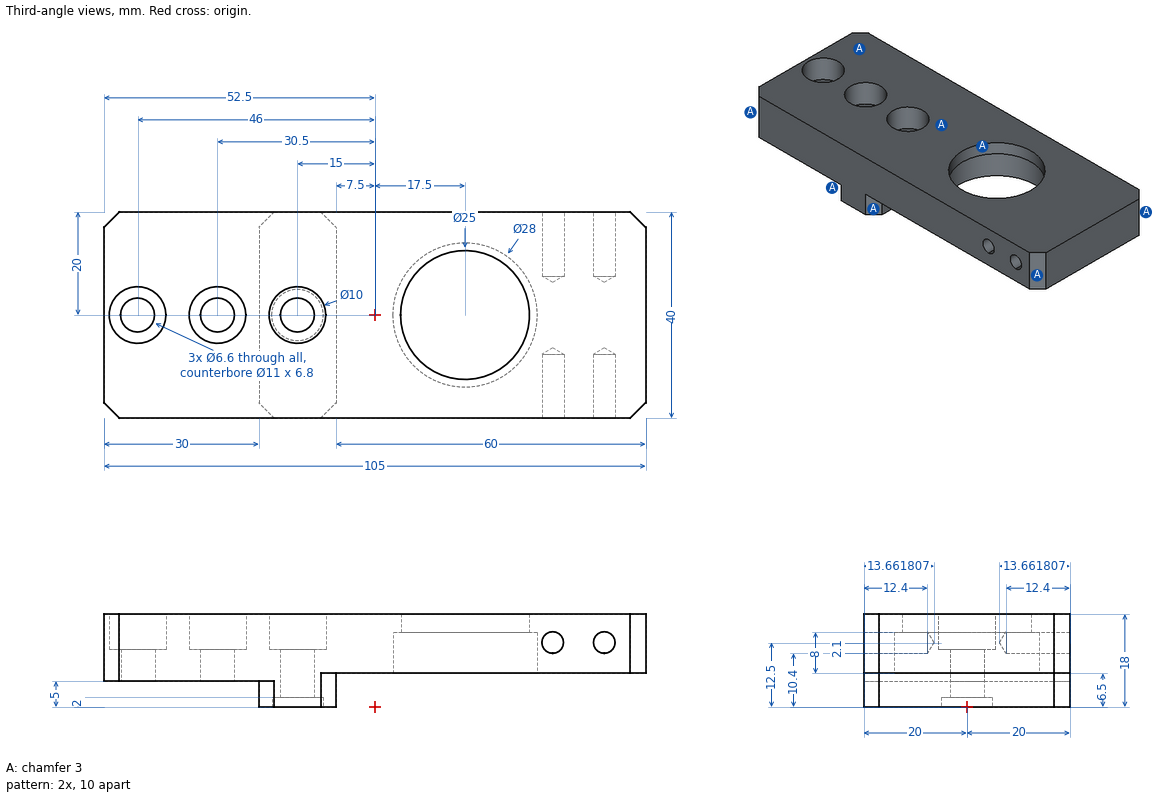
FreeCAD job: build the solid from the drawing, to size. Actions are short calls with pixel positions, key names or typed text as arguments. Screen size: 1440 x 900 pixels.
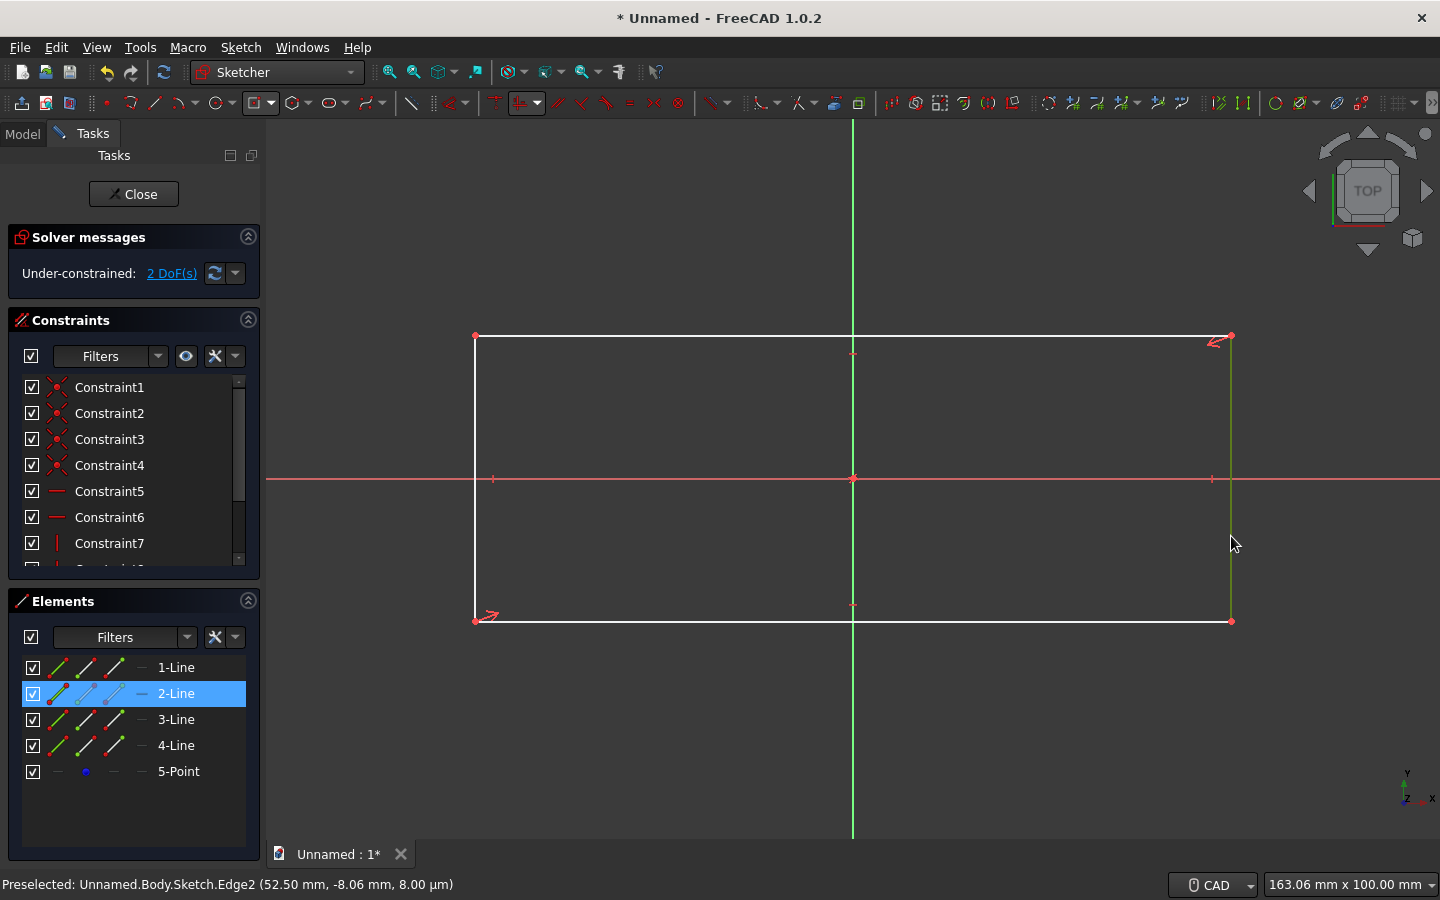
click(468, 104)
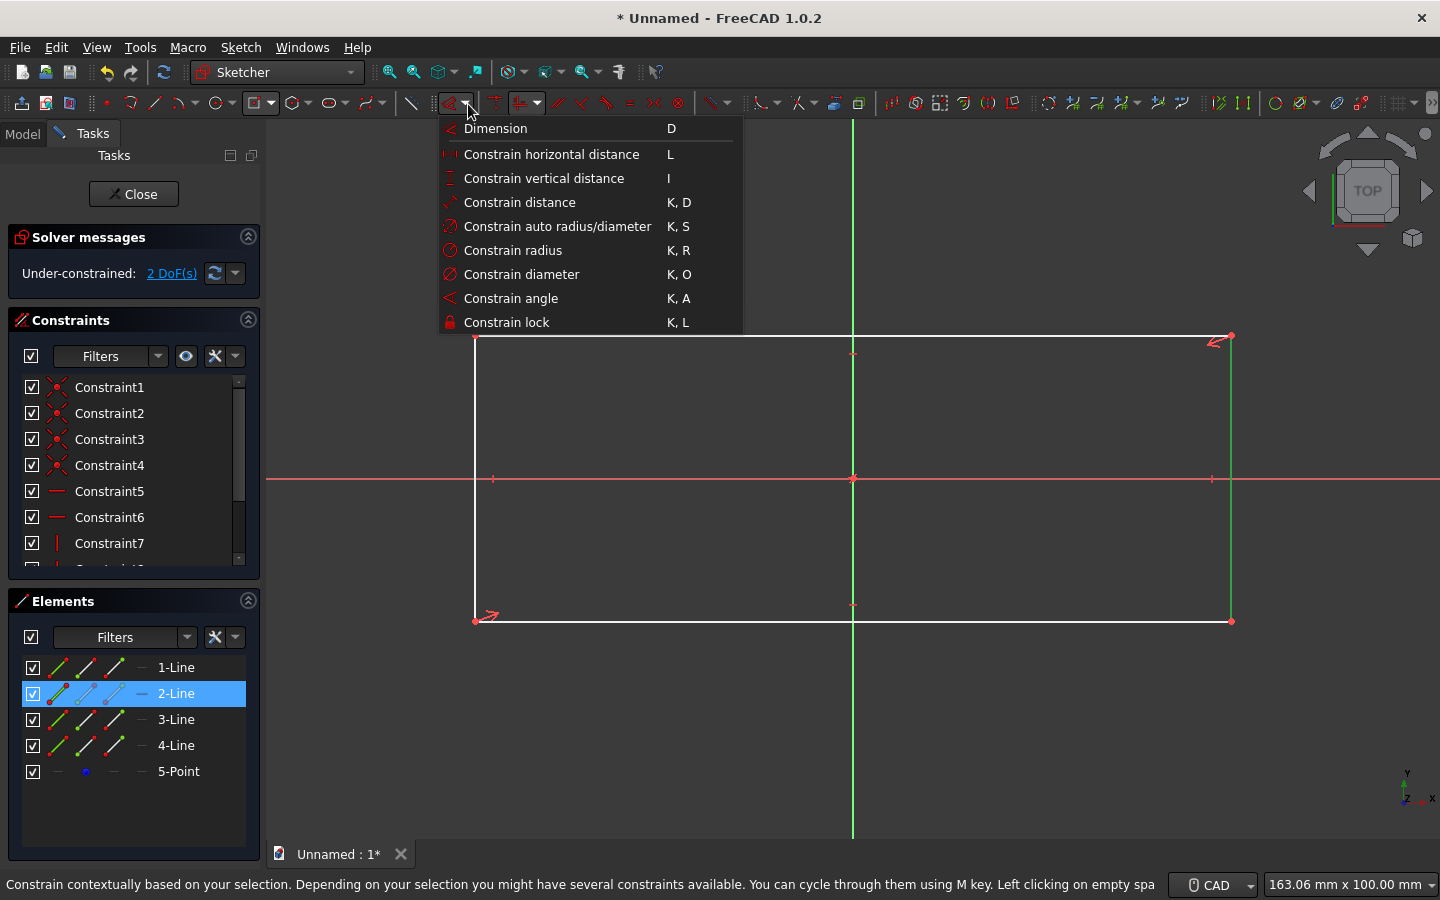
click(591, 178)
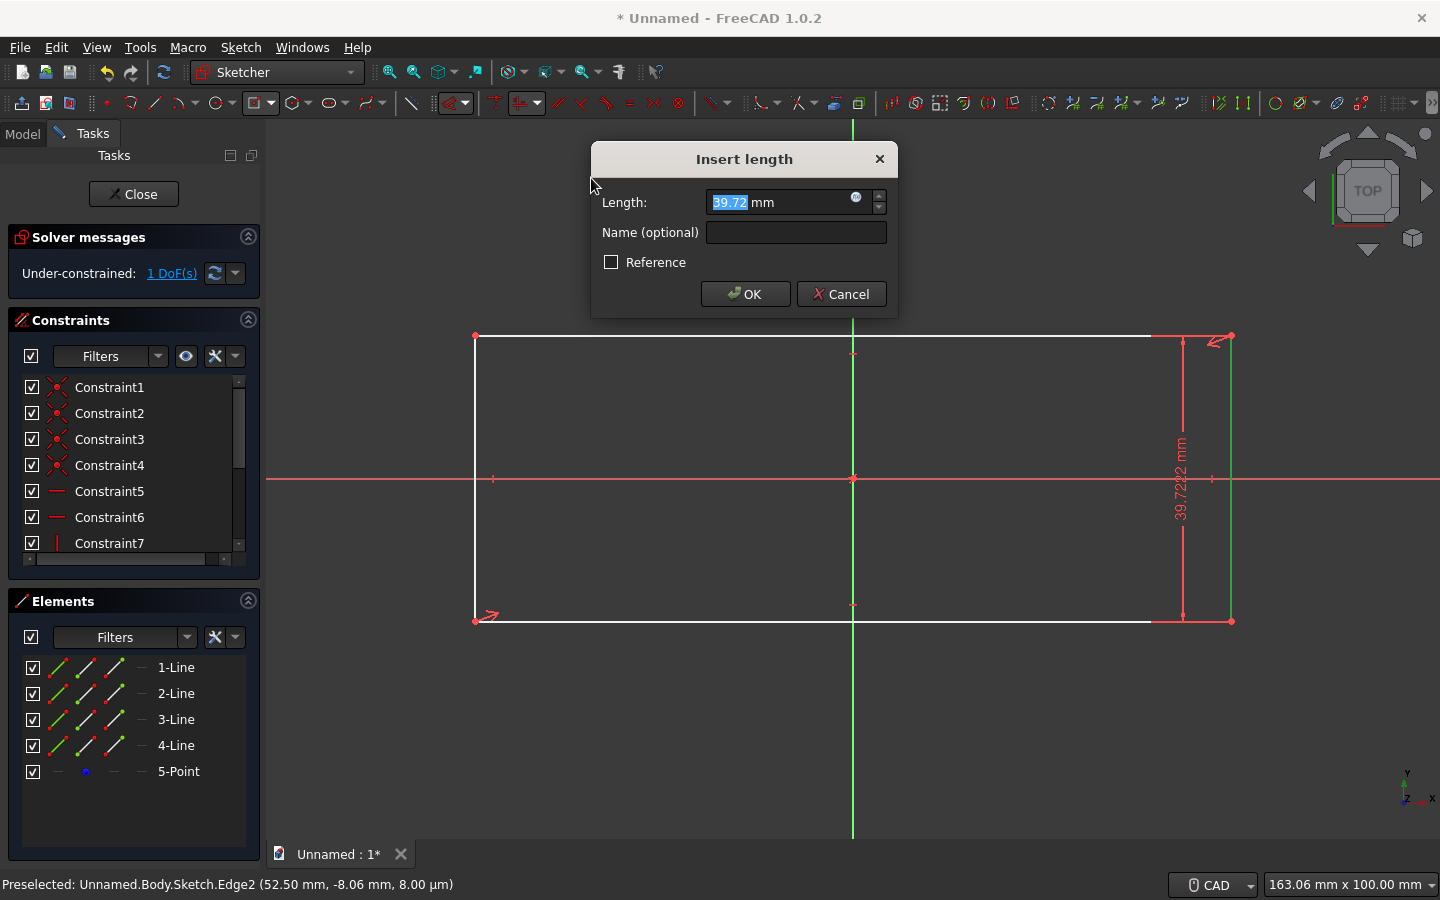
text(40)
key(Return)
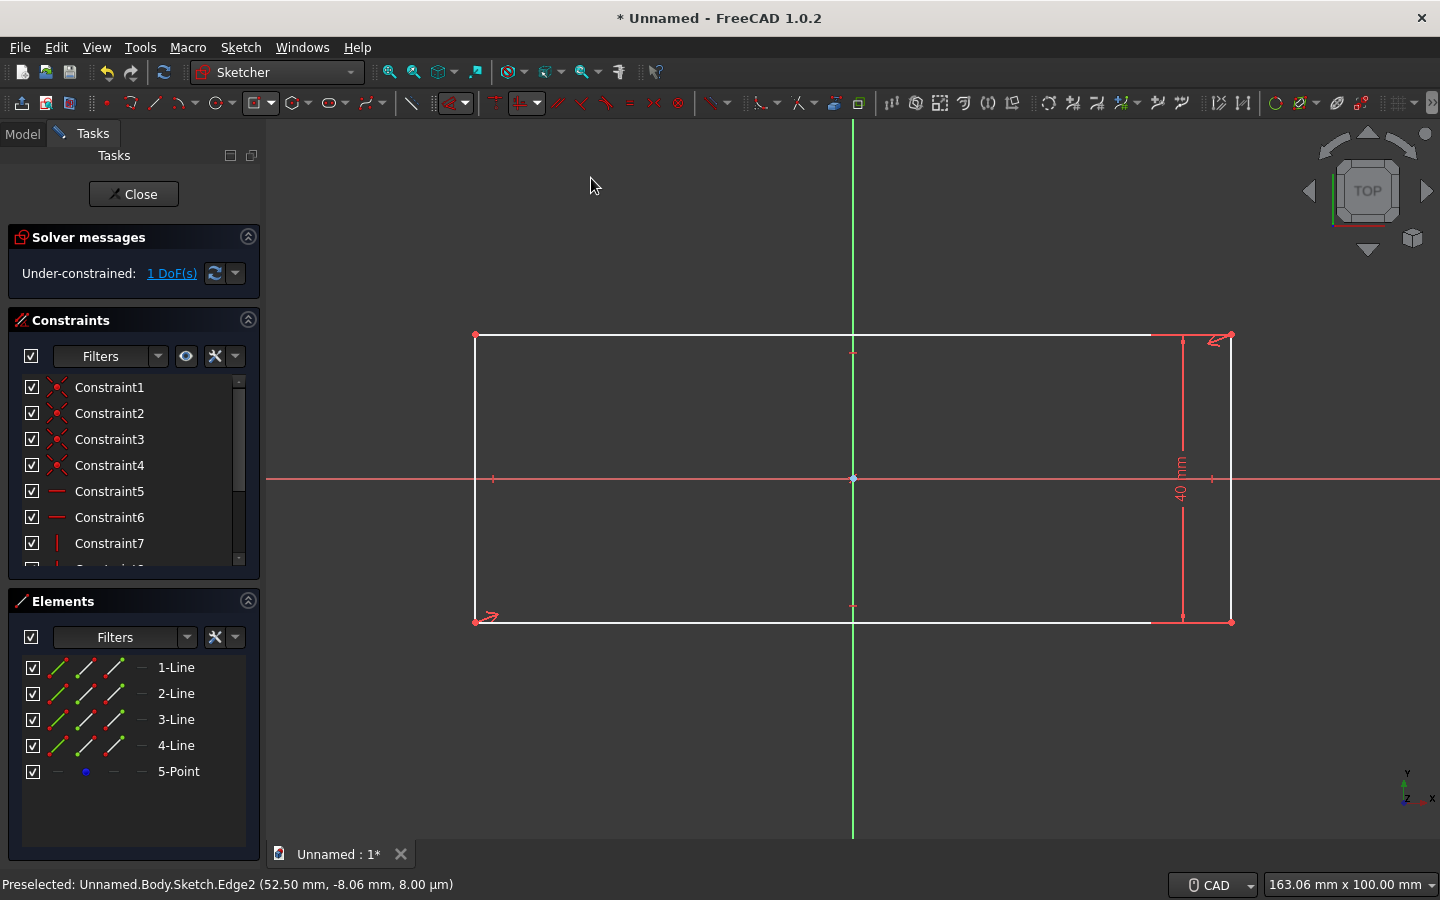
click(702, 623)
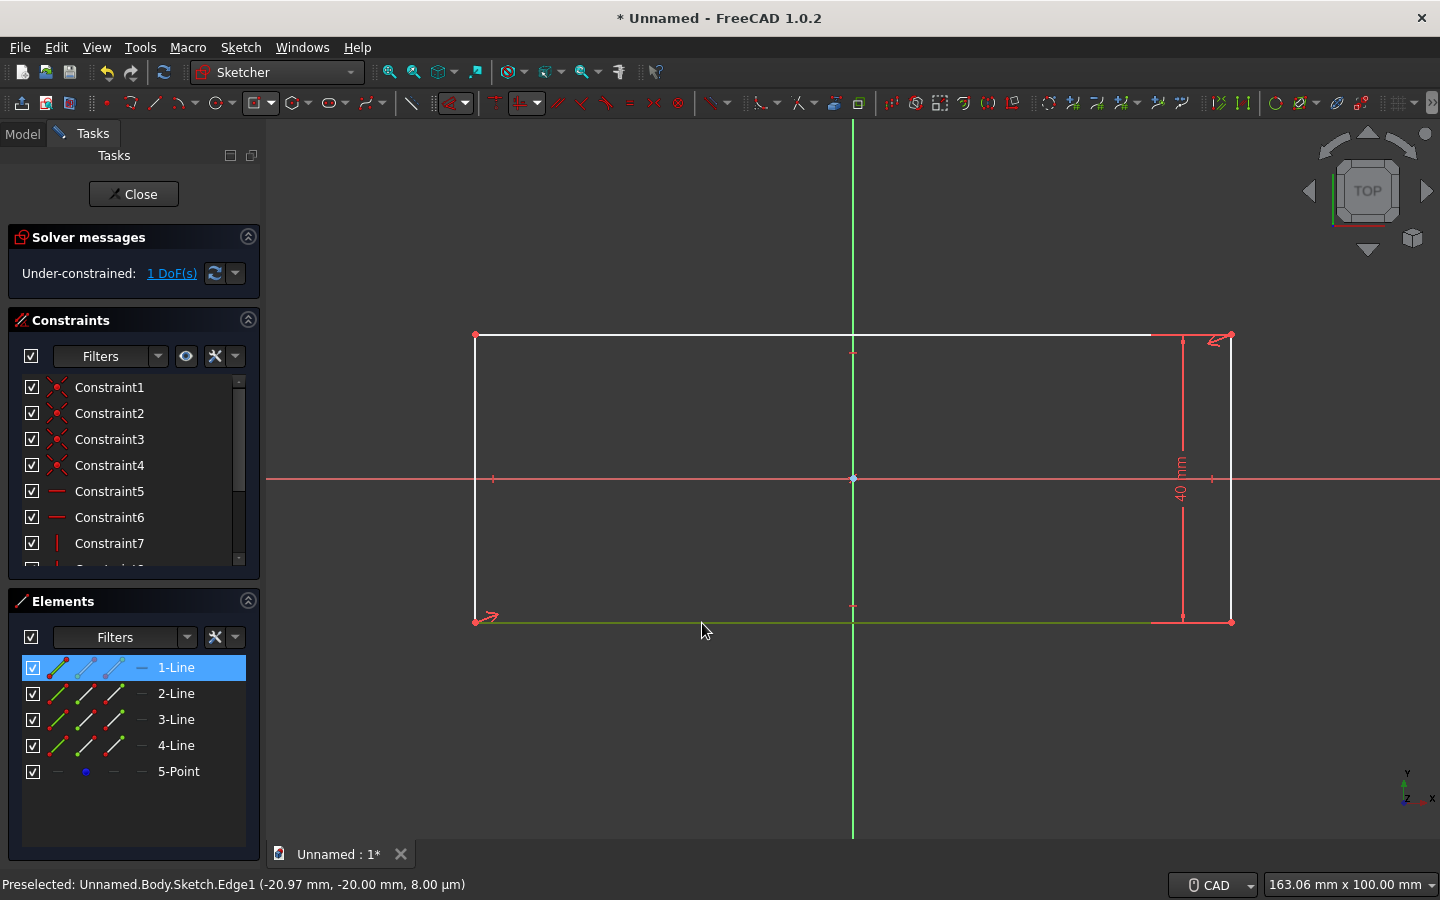
click(468, 104)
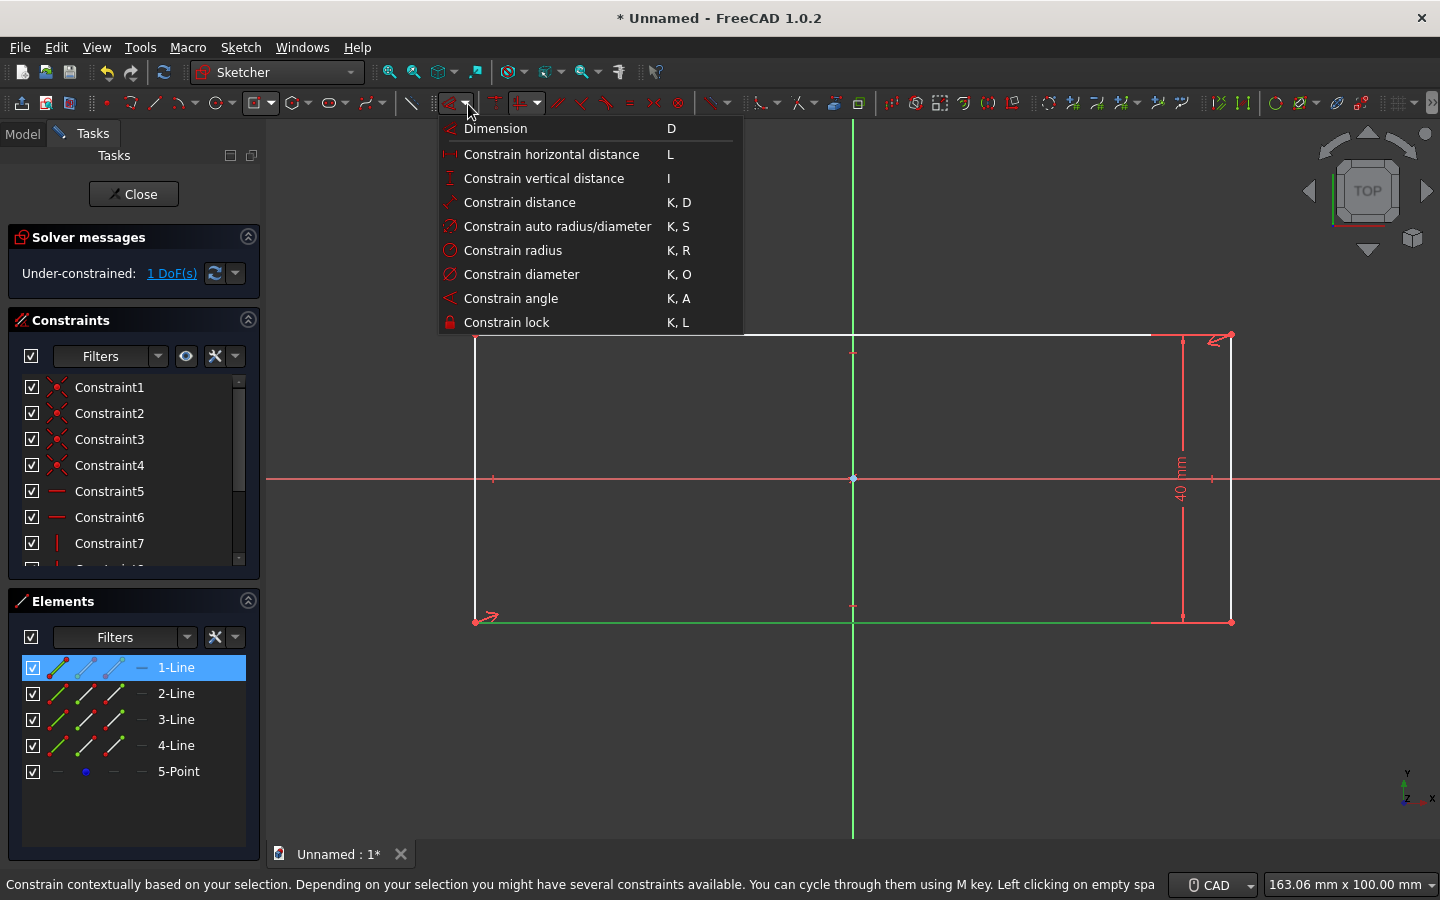
click(591, 154)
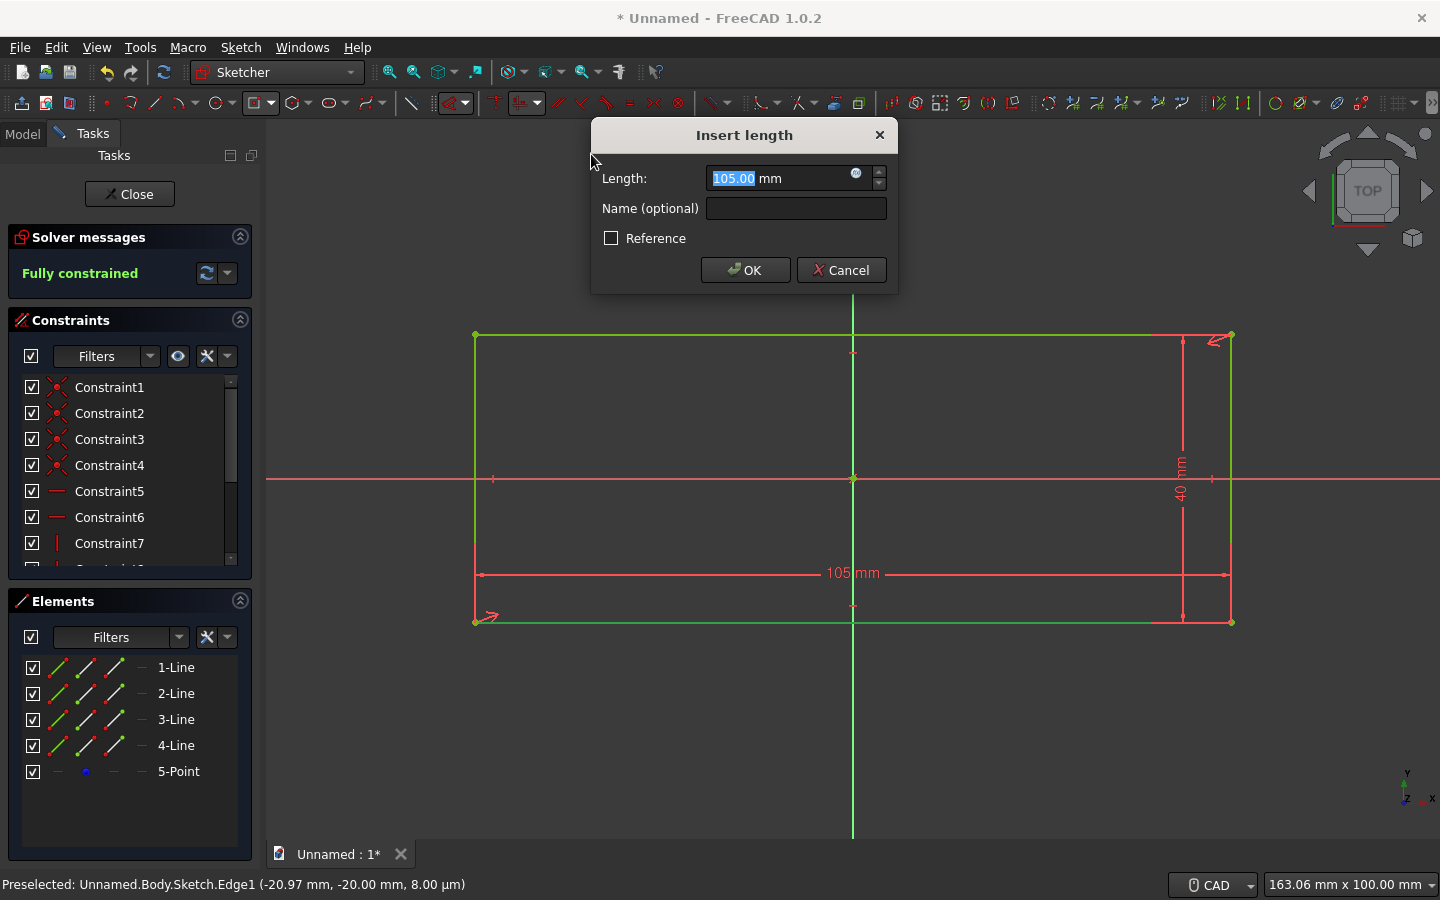
text(105)
key(Return)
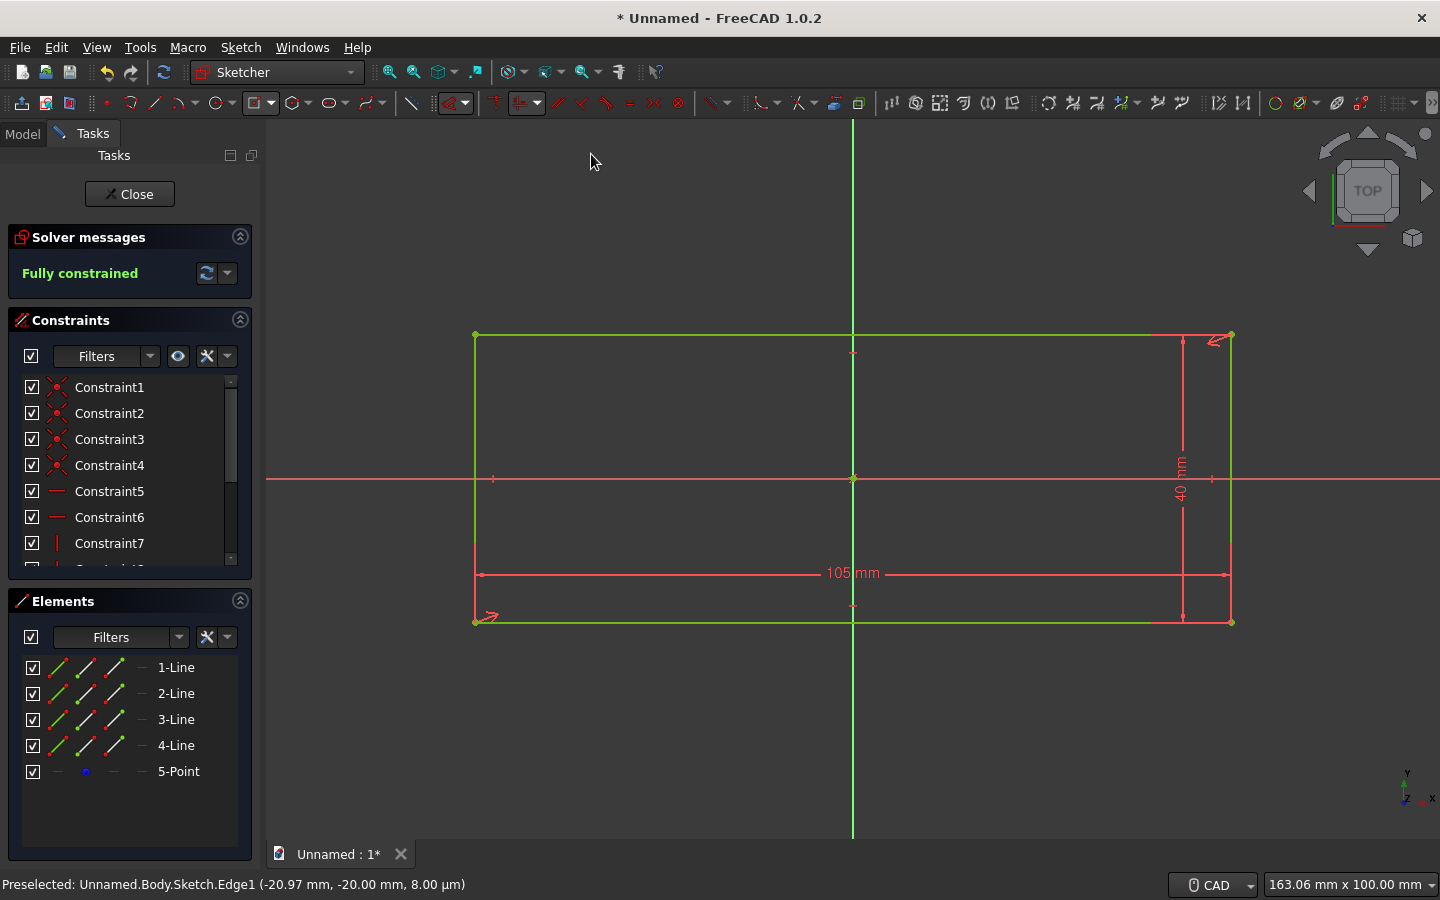
click(130, 194)